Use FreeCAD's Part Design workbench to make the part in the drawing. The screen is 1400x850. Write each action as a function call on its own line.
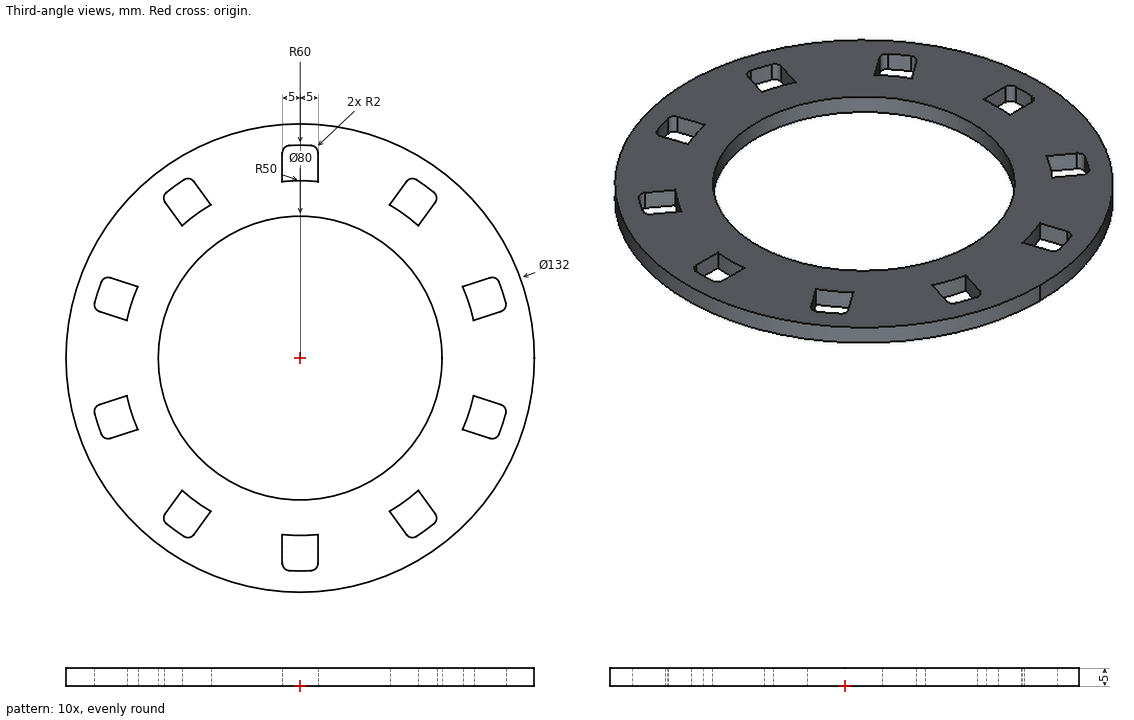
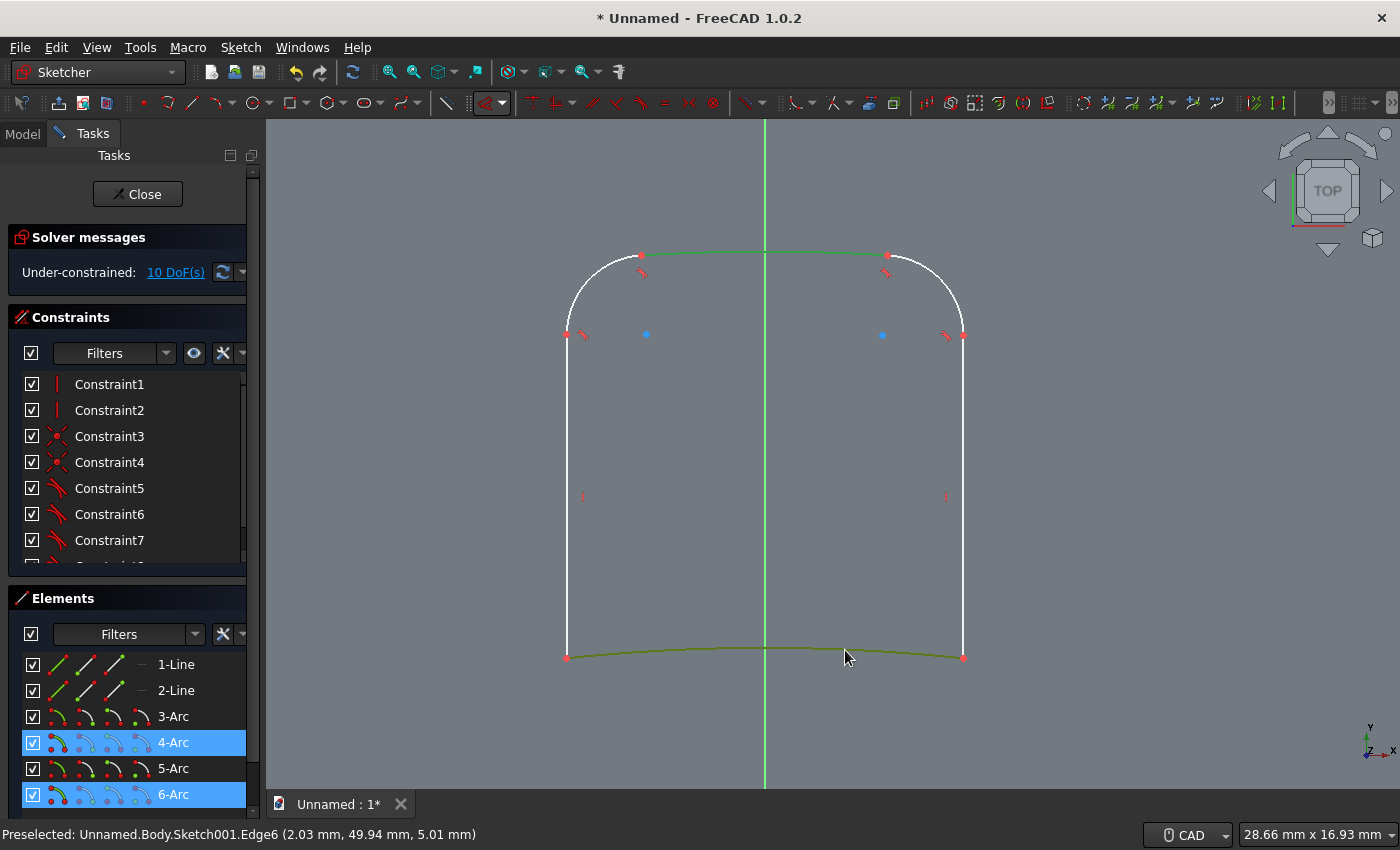
key(c)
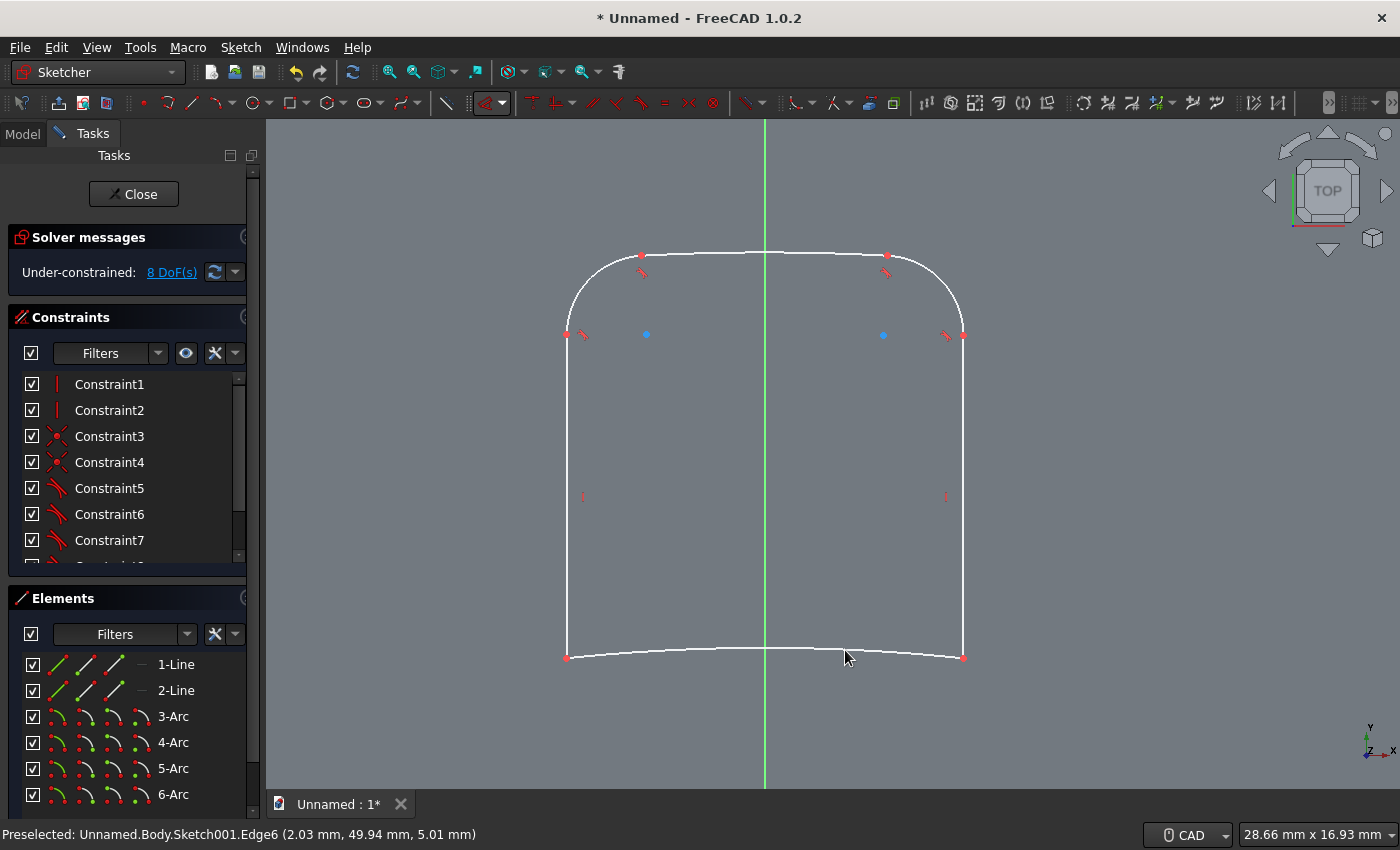
scroll(764, 210, down, 8)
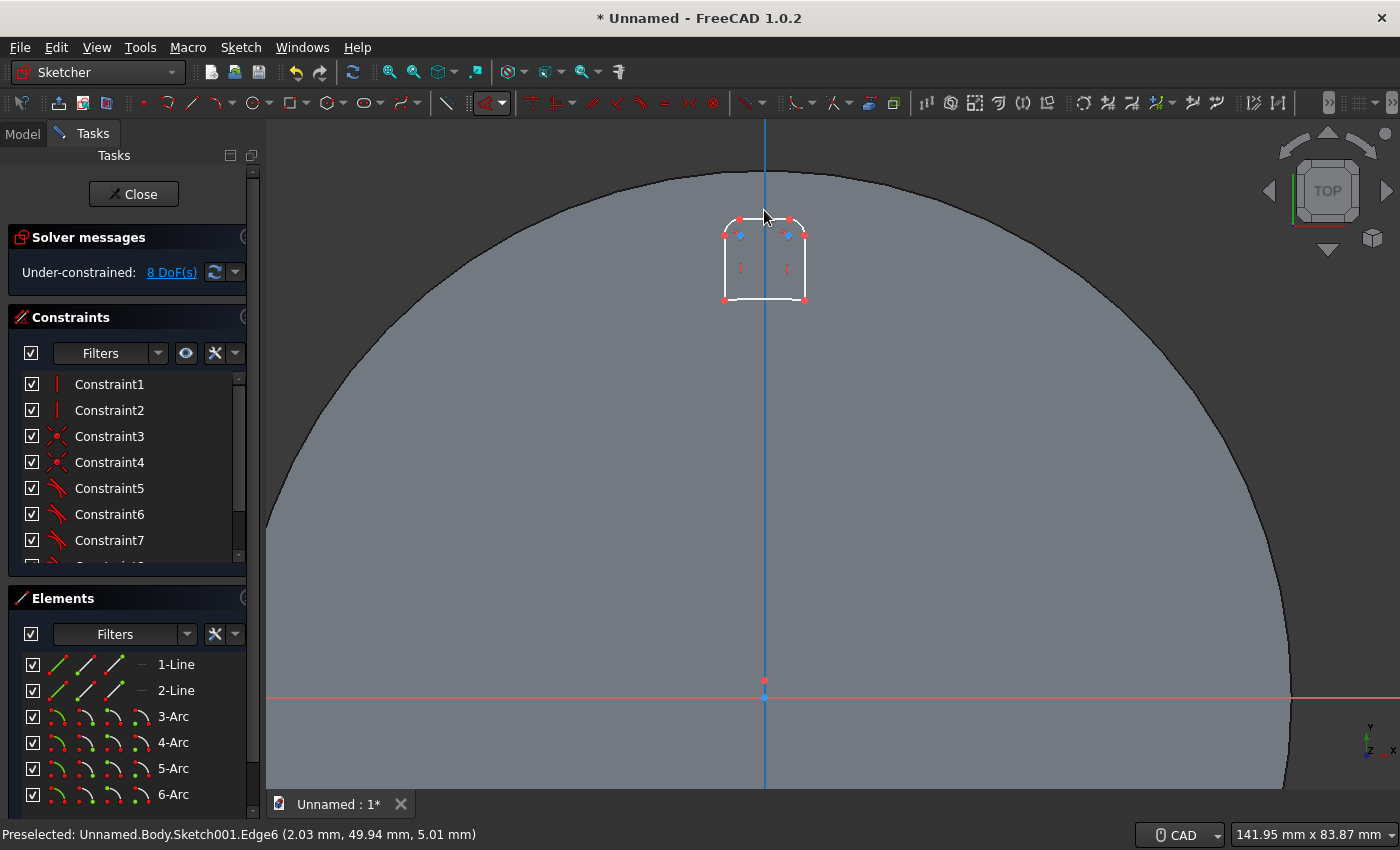
scroll(765, 689, up, 5)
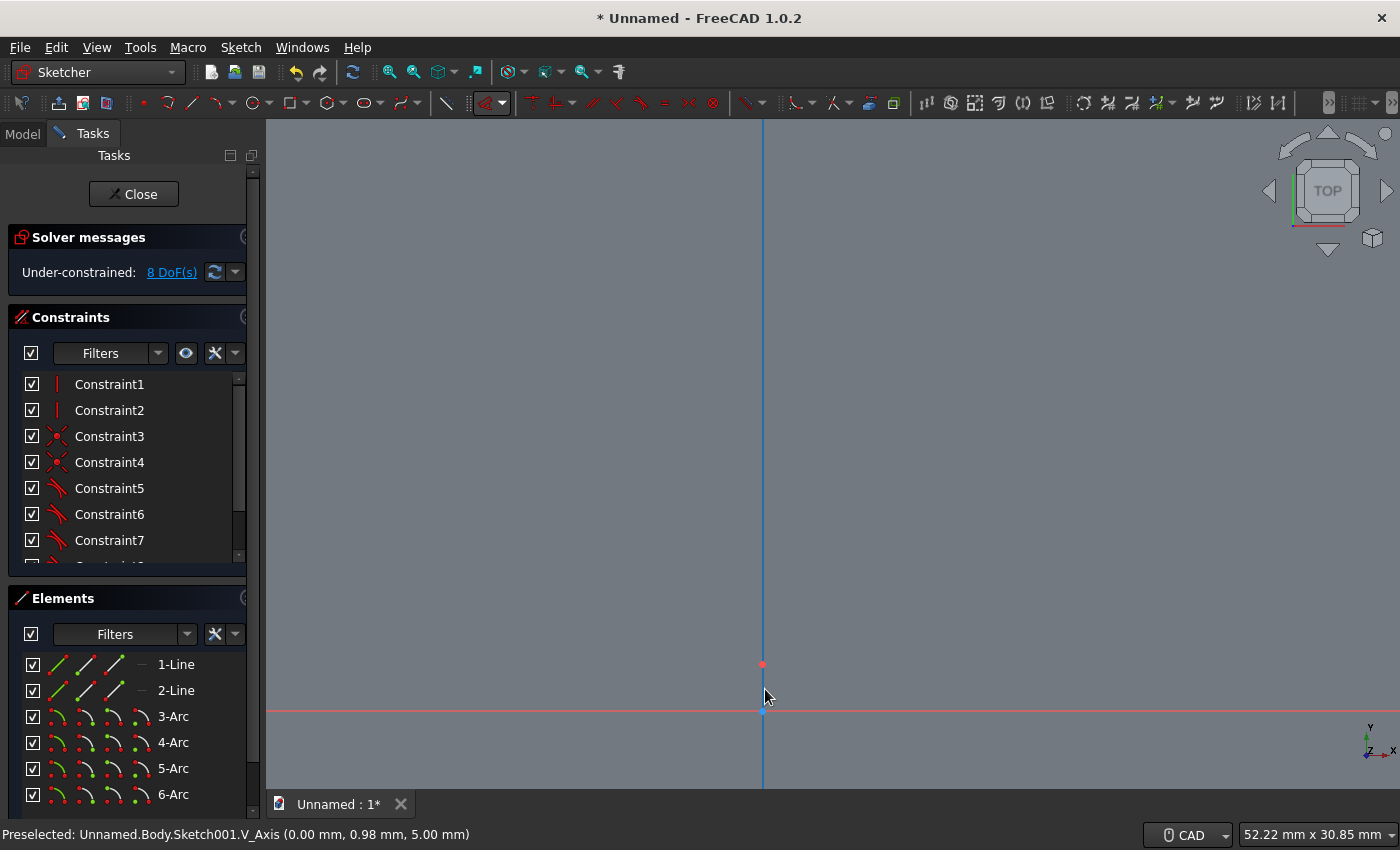
drag(753, 655, 773, 721)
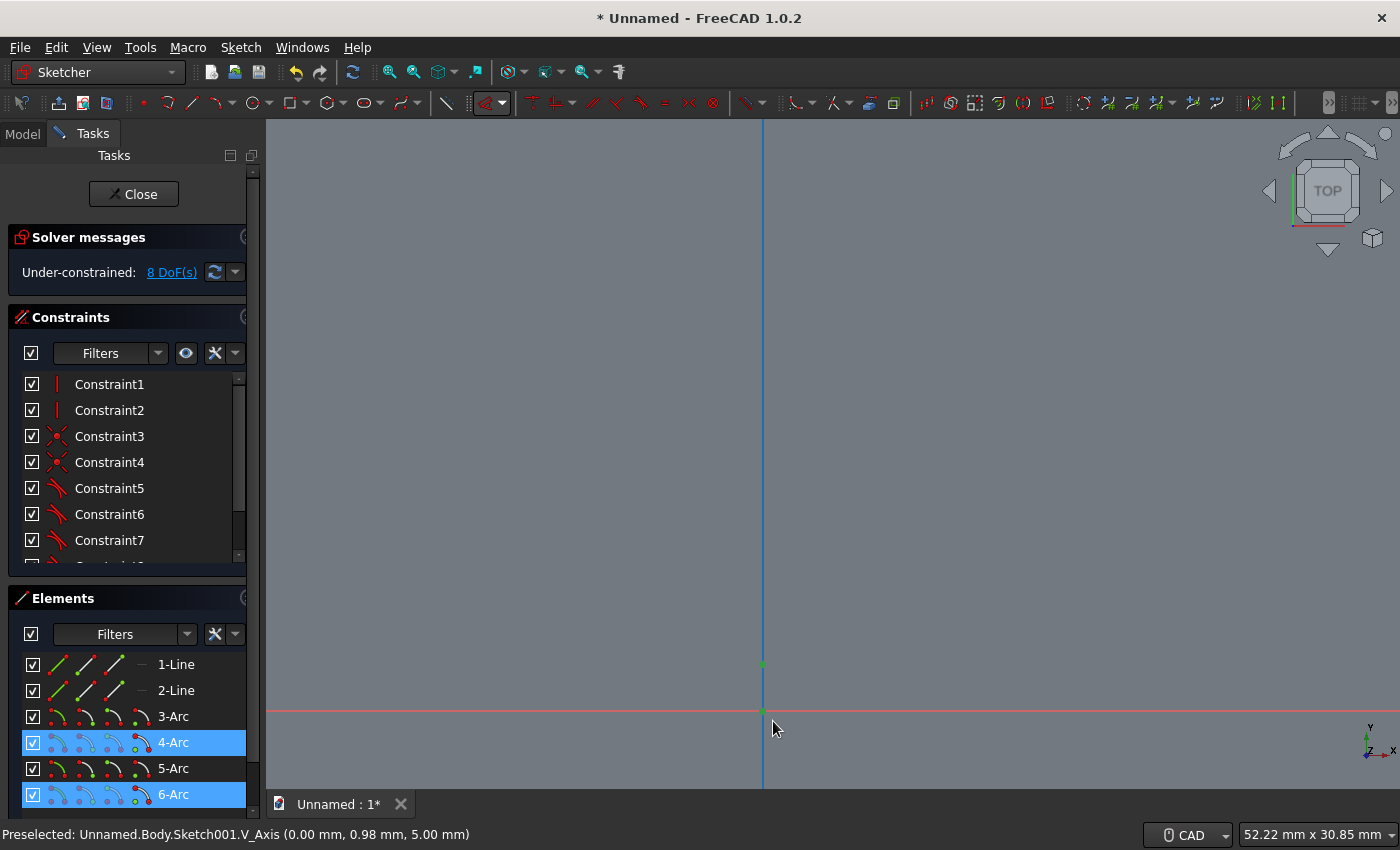
key(c)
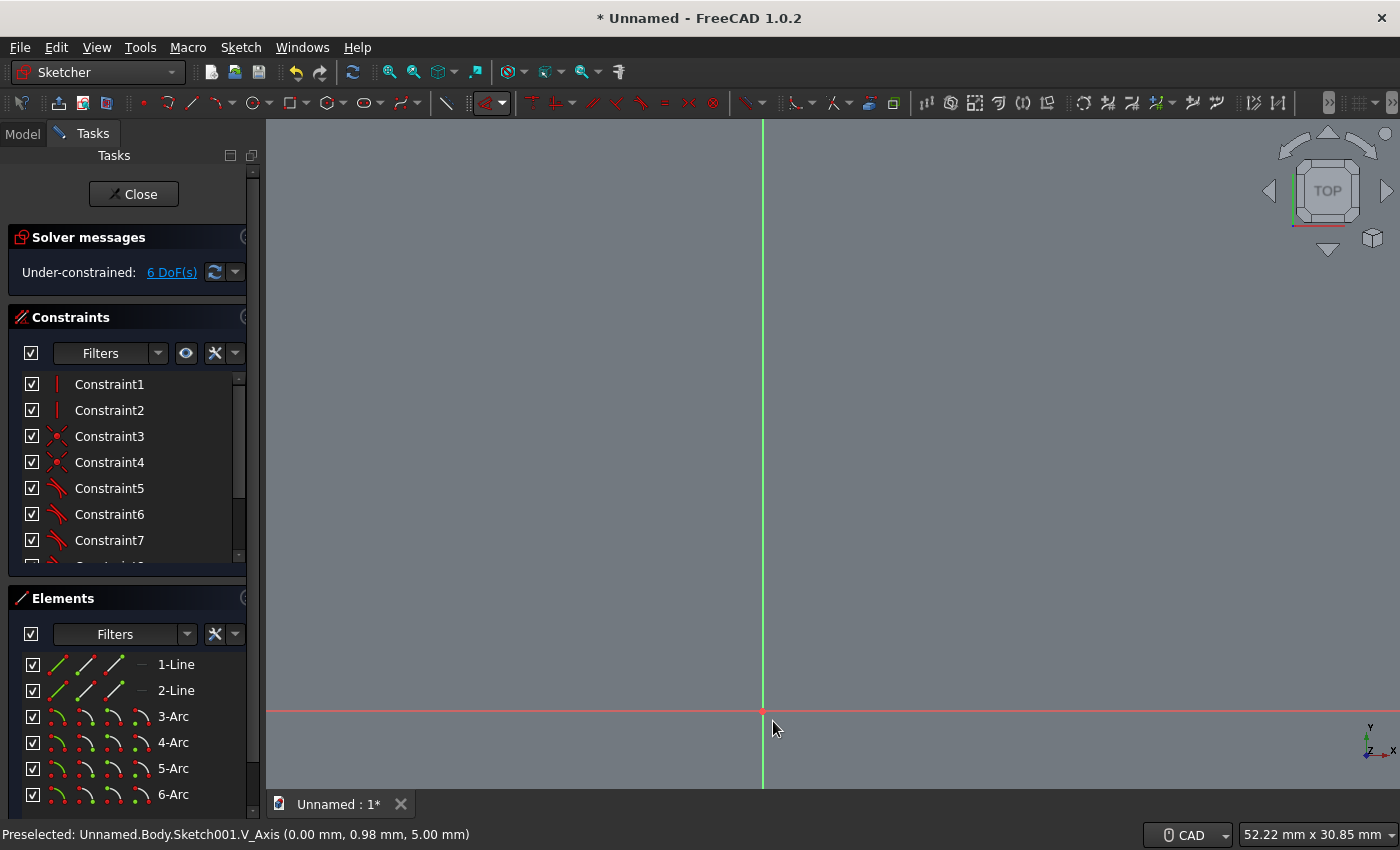
scroll(764, 454, down, 5)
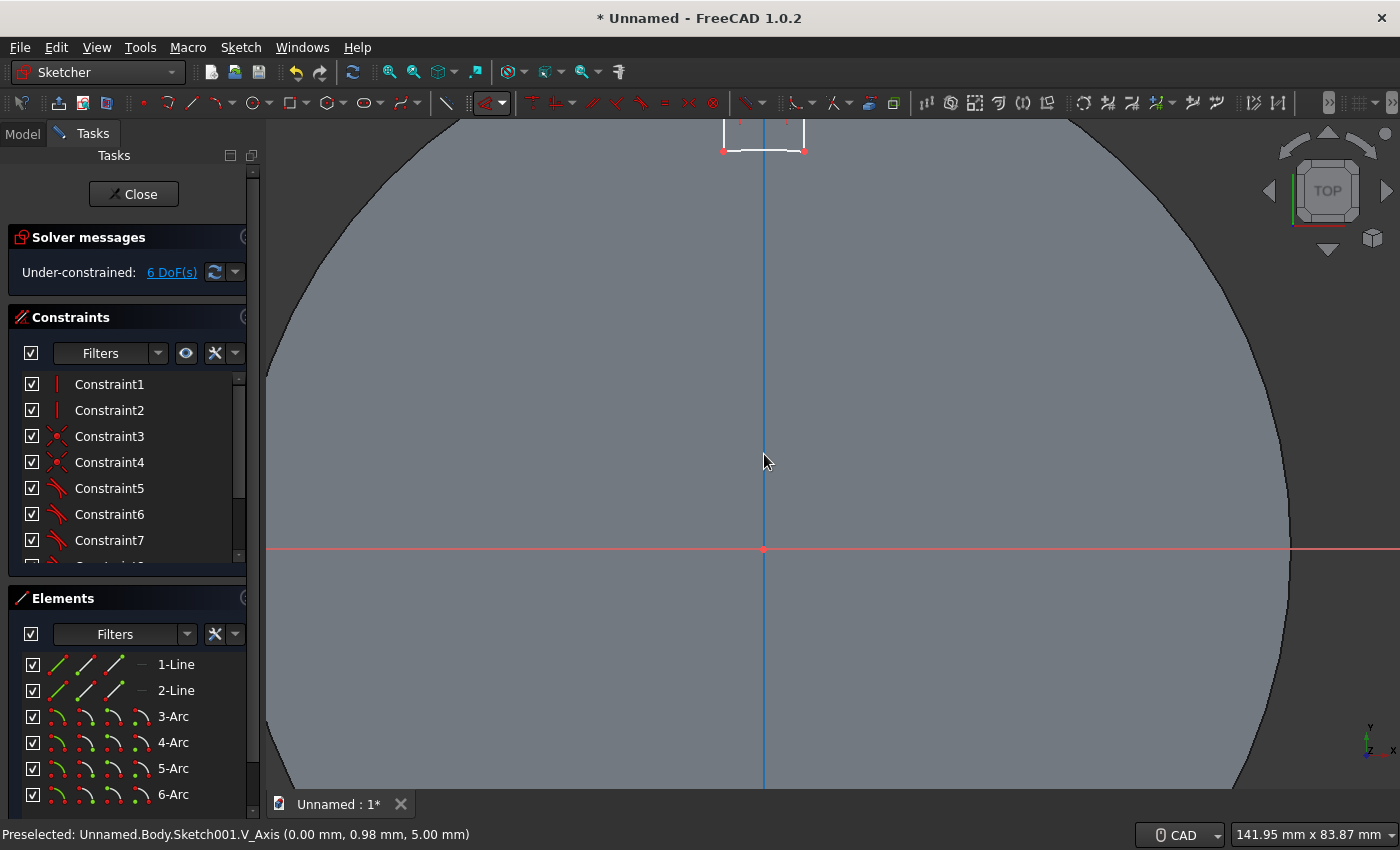
scroll(764, 454, down, 5)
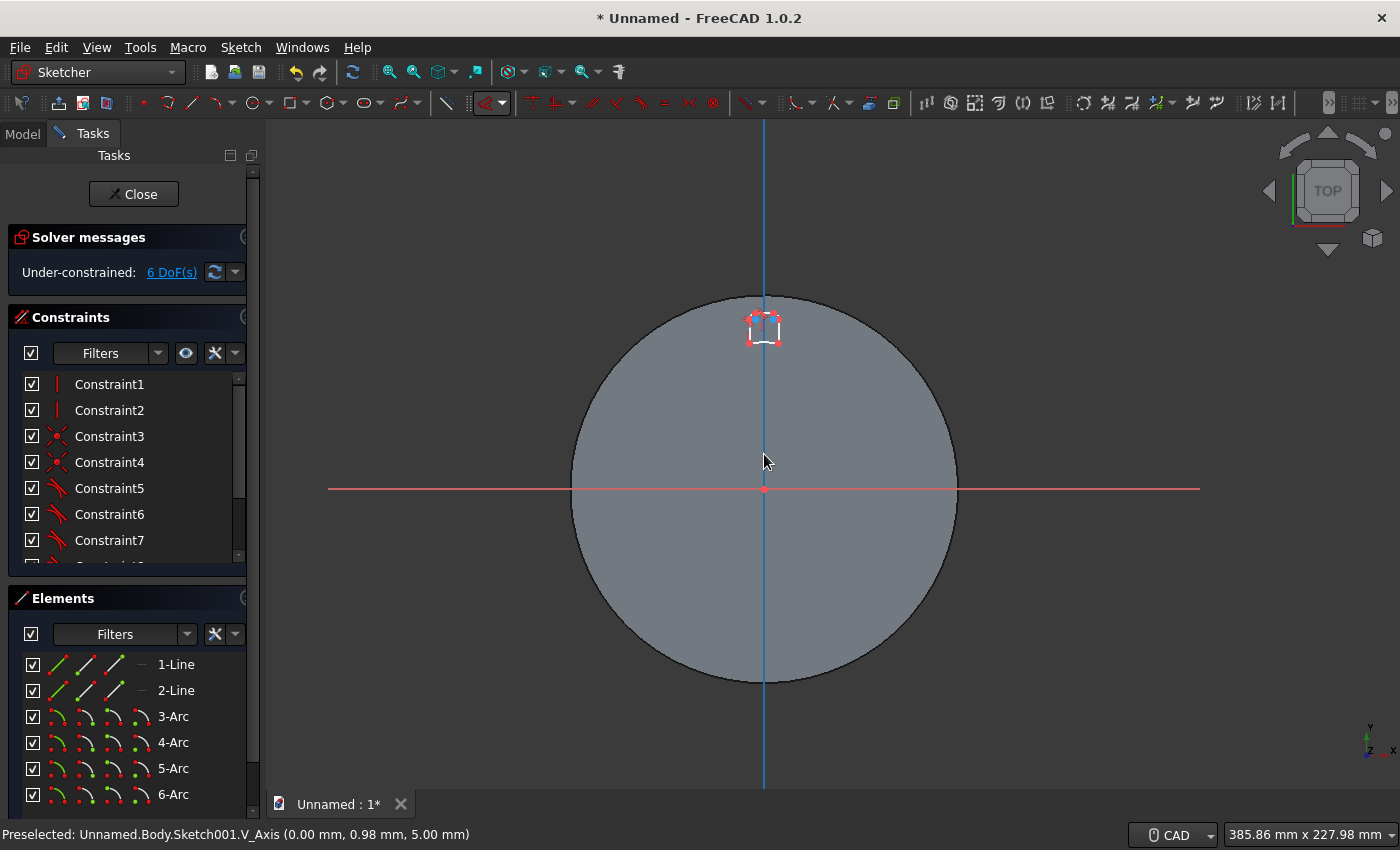
scroll(764, 318, up, 13)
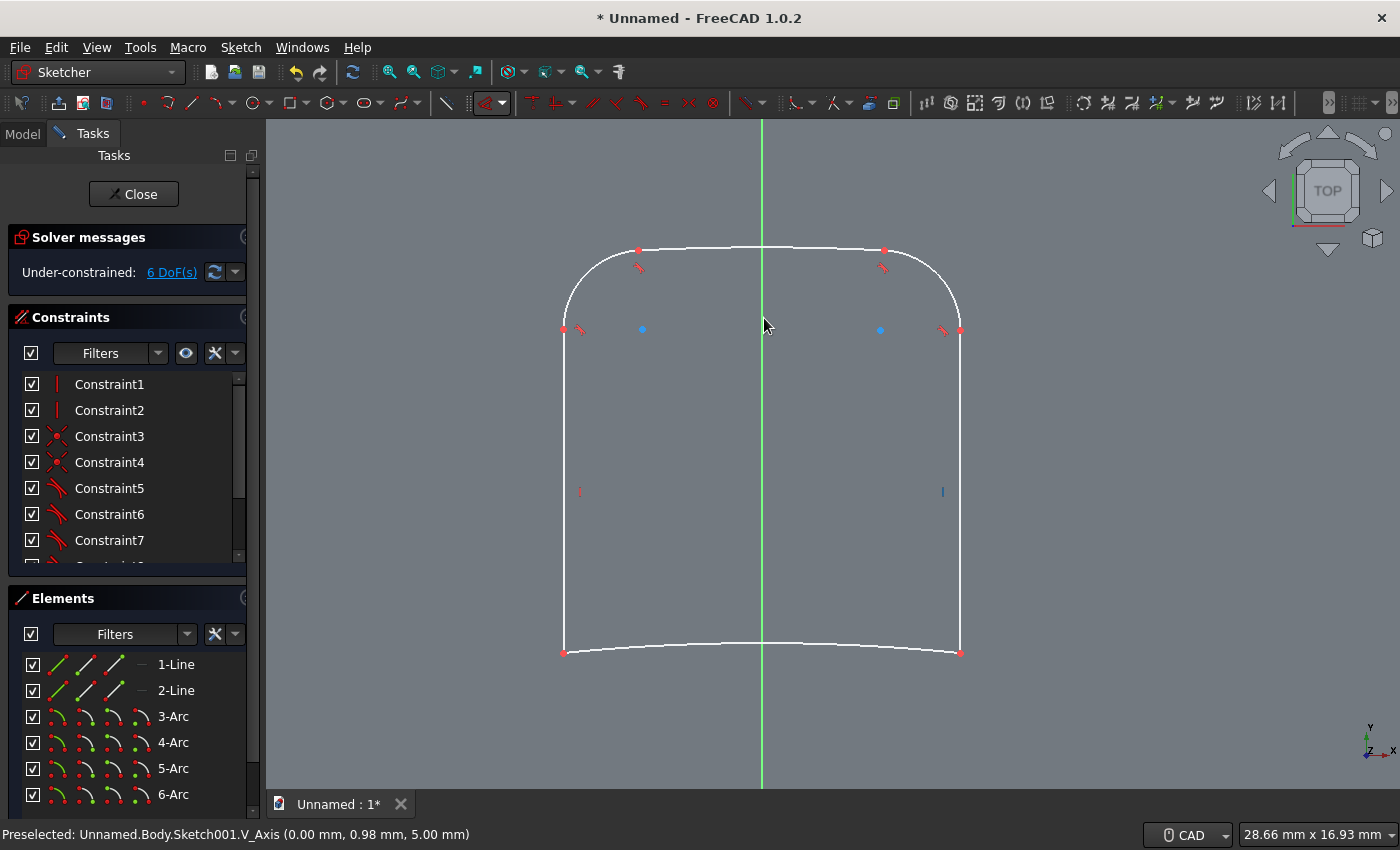
click(952, 295)